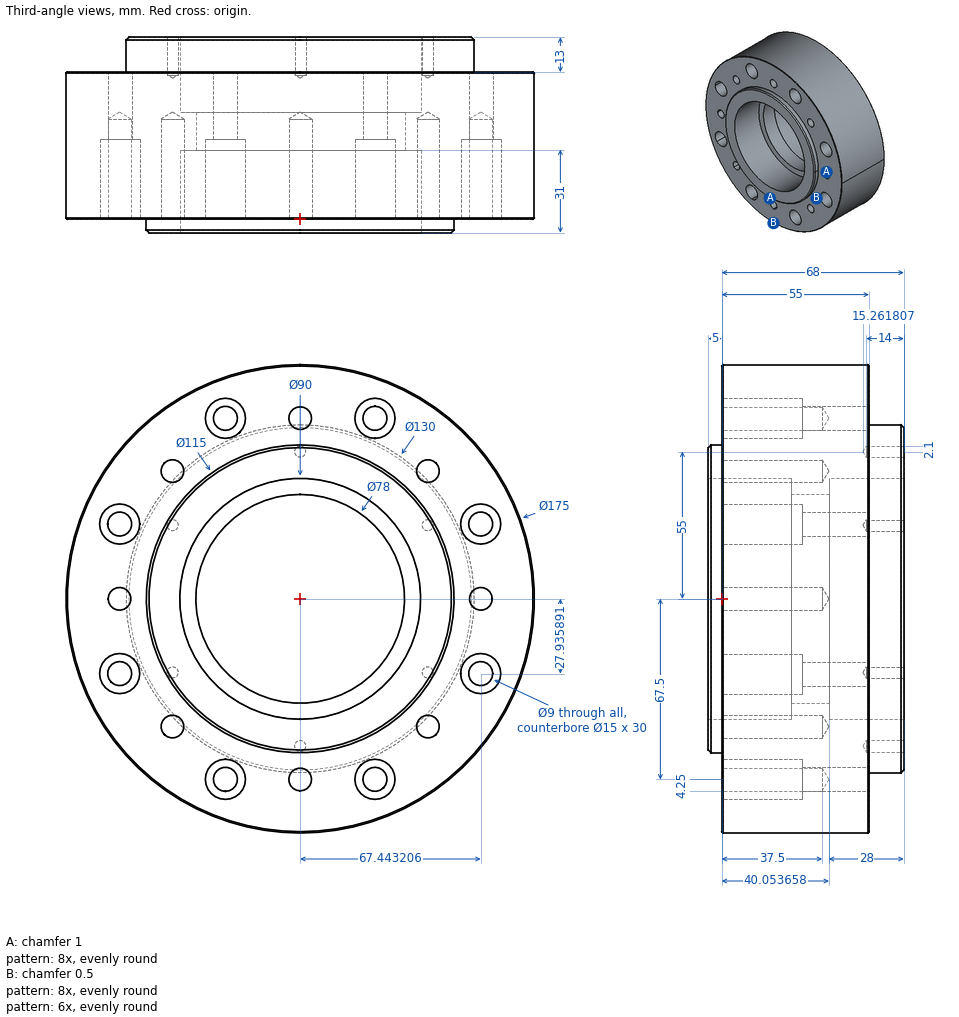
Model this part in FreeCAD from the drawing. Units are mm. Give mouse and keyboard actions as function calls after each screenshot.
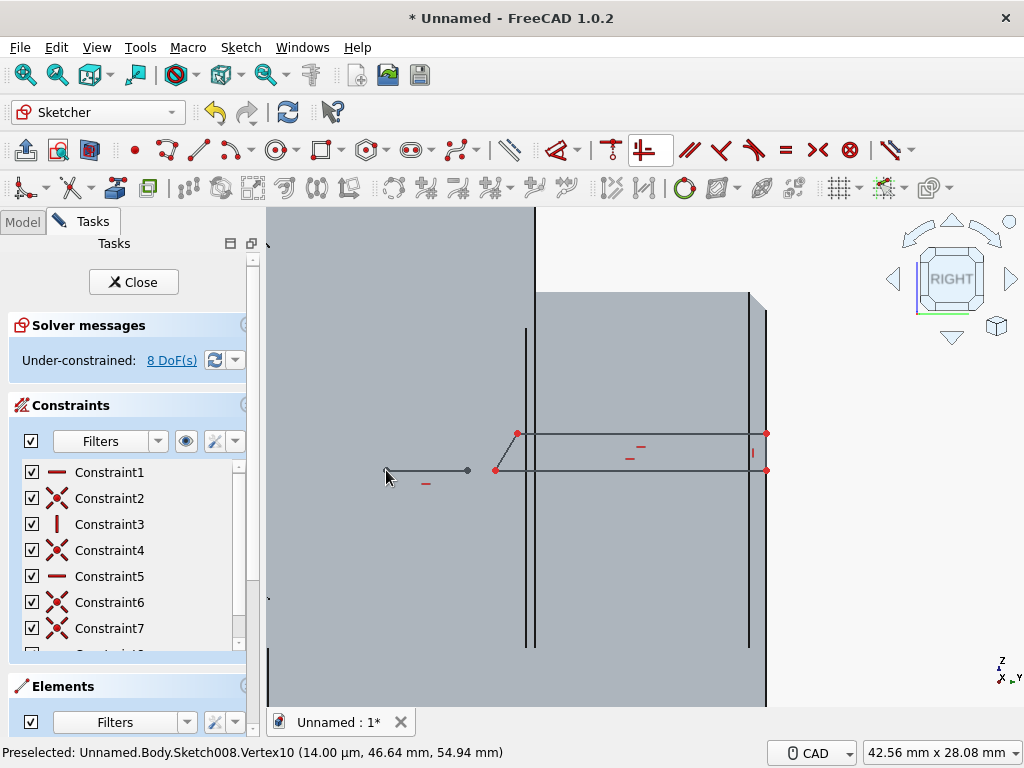
click(443, 471)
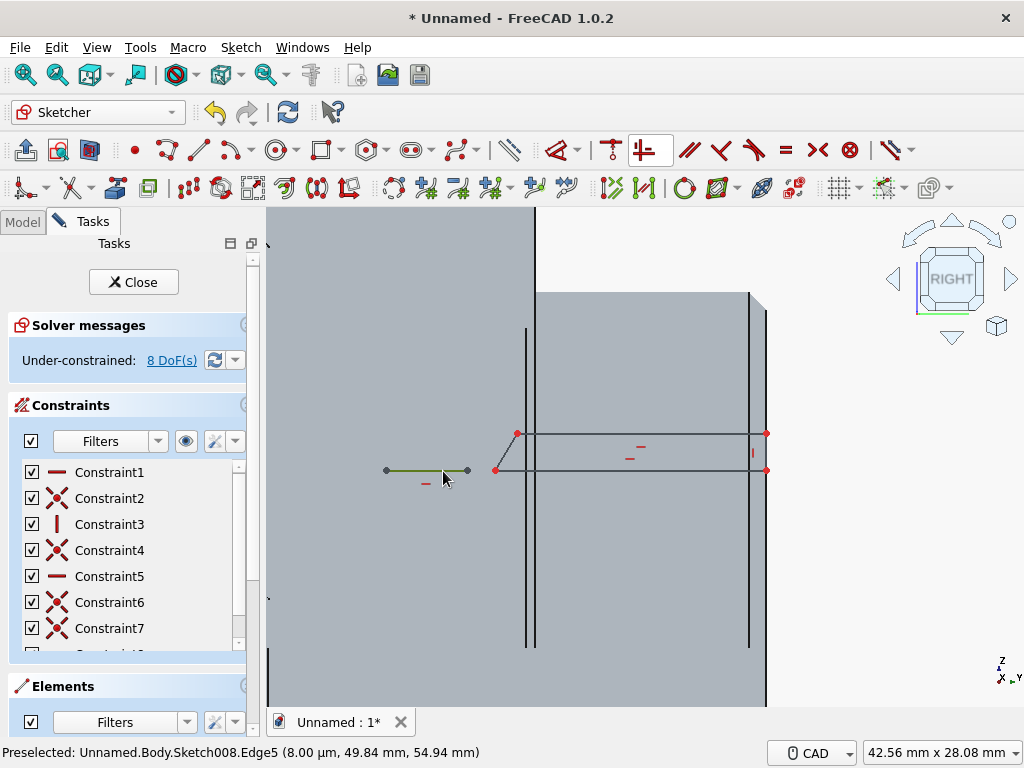
click(510, 150)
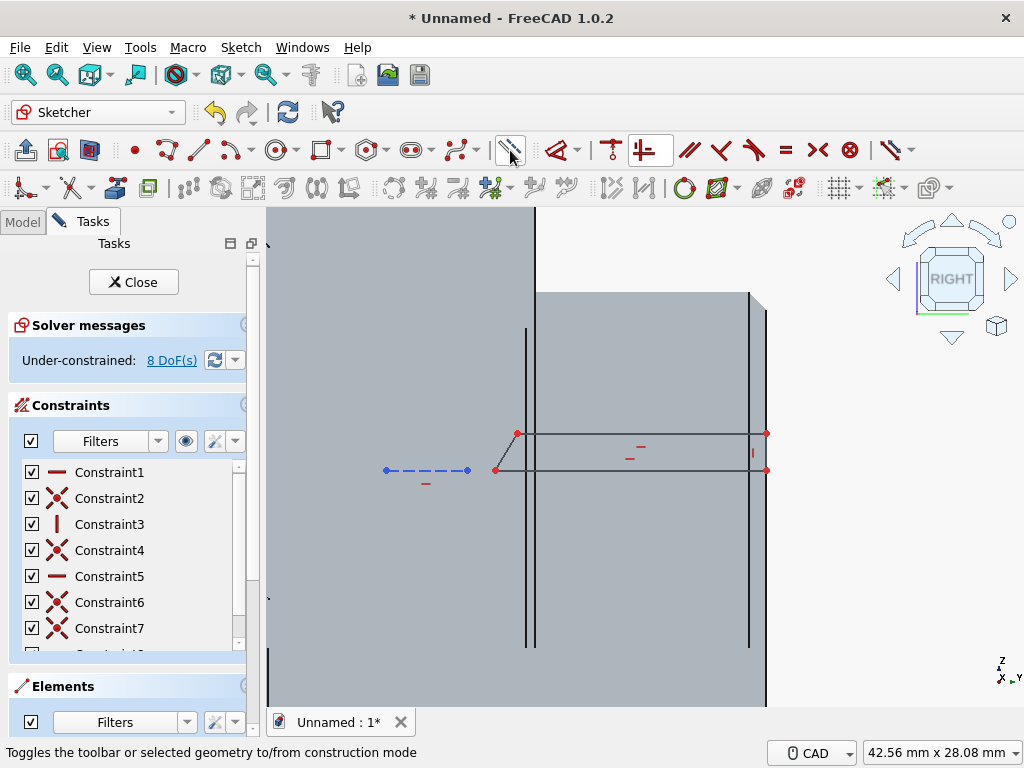
click(556, 150)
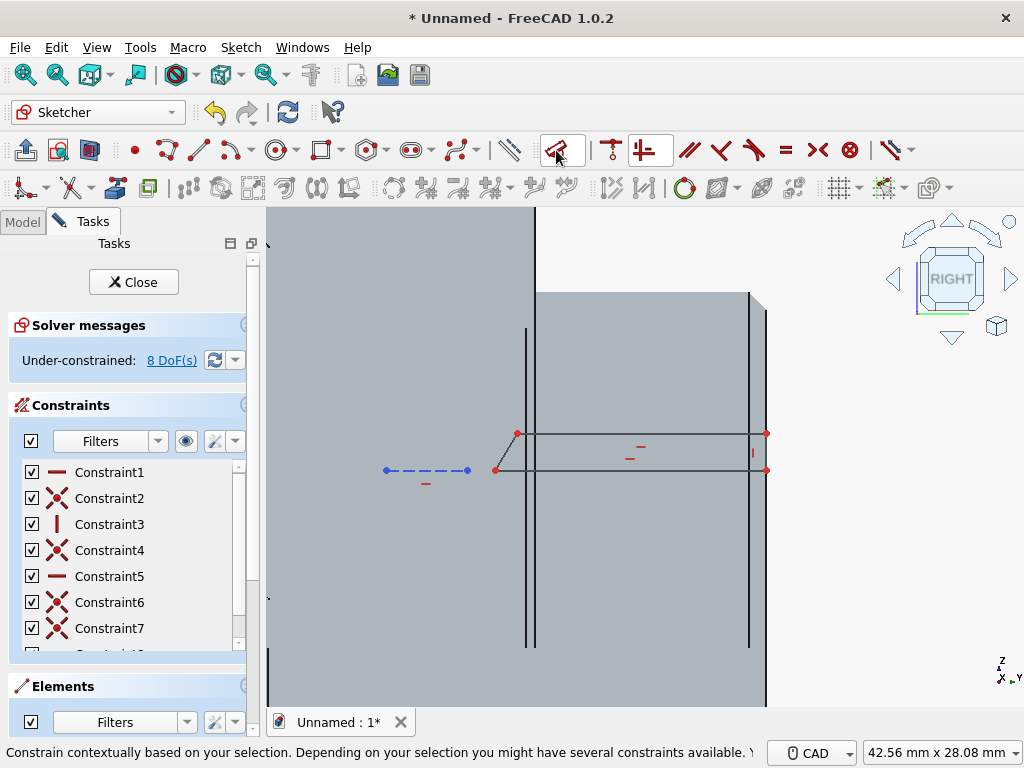
click(691, 434)
click(642, 400)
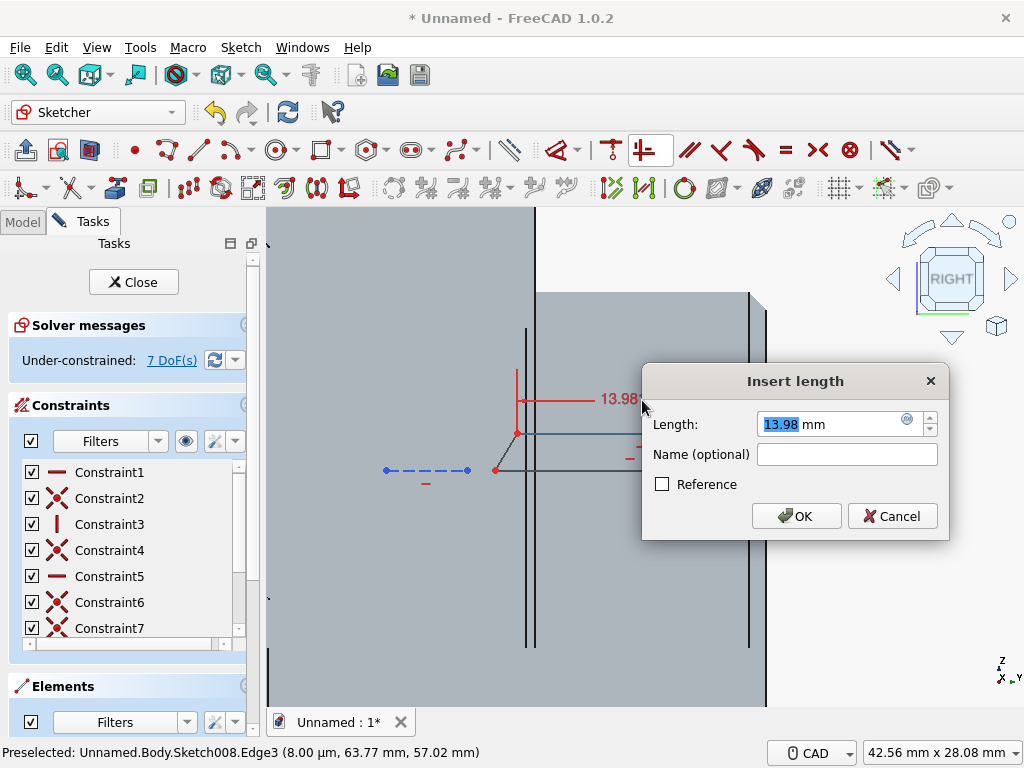
text(14)
key(Return)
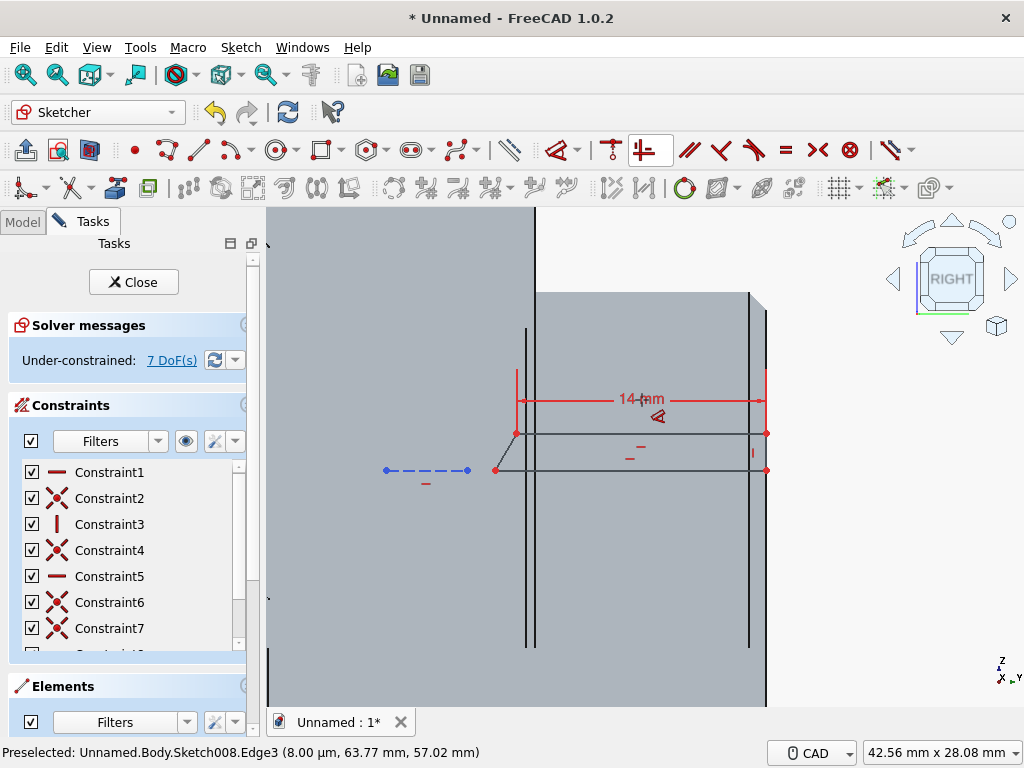
scroll(766, 460, up, 2)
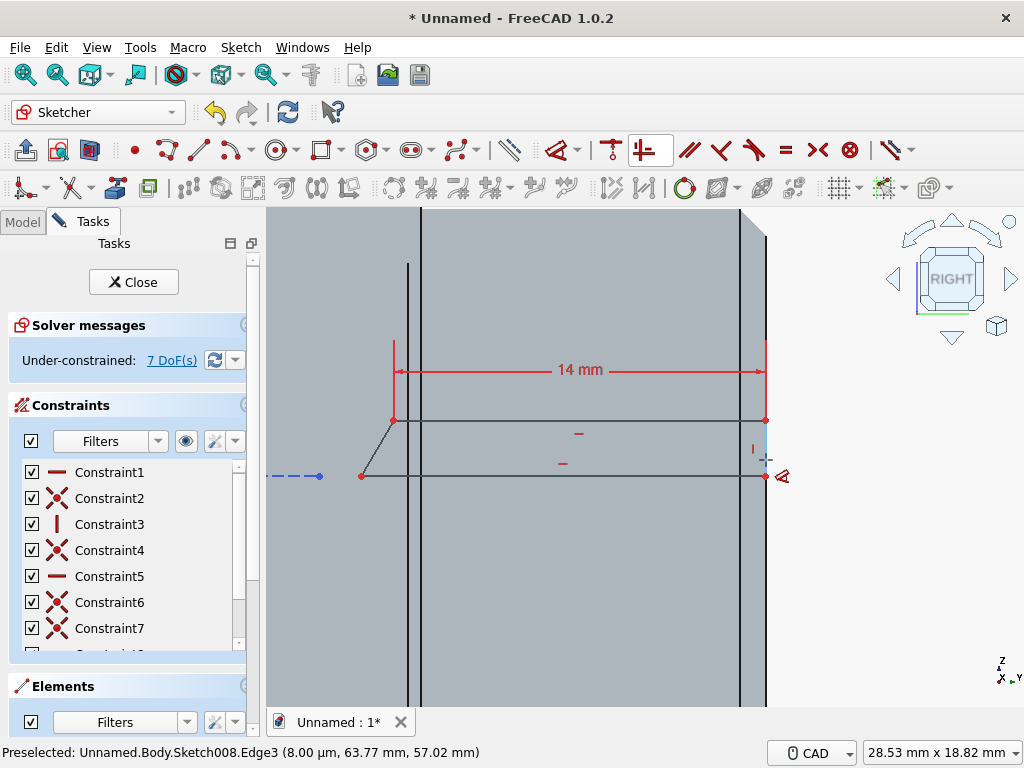
click(766, 460)
click(800, 449)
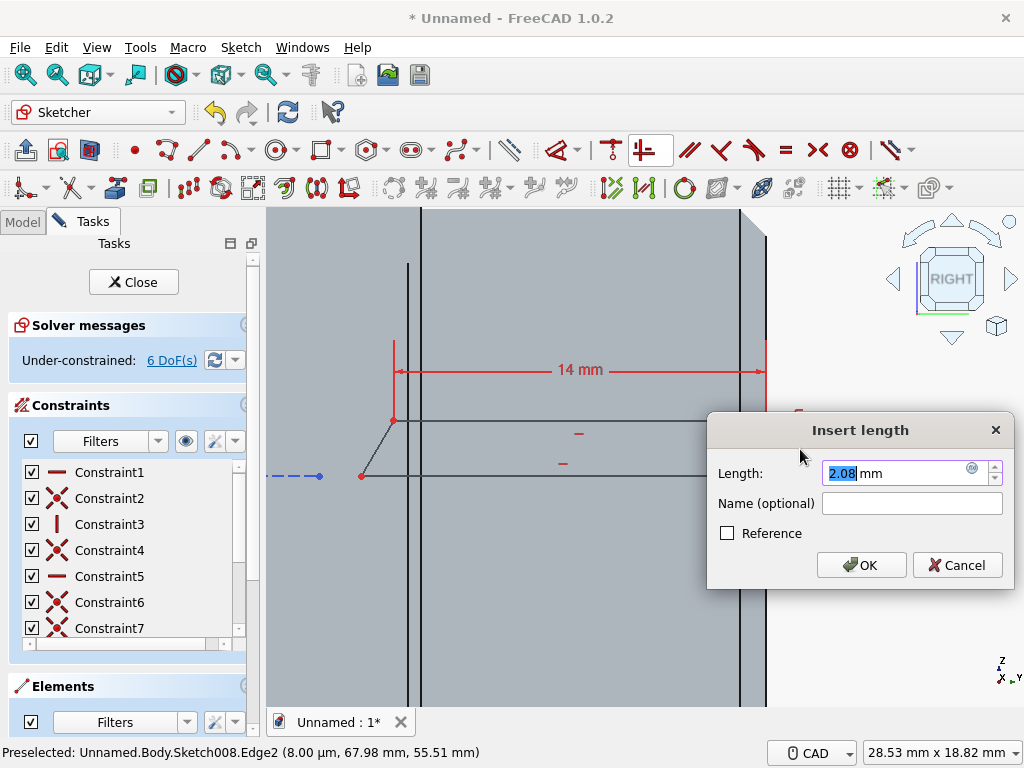
text(2.1)
key(Return)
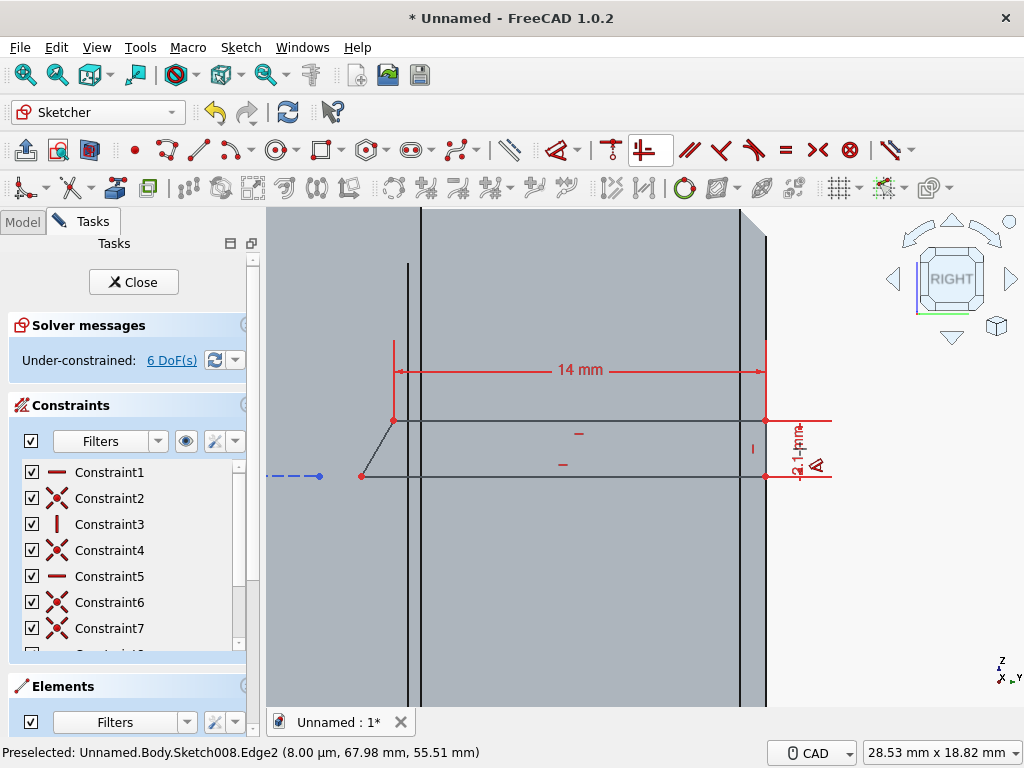
click(361, 477)
click(395, 578)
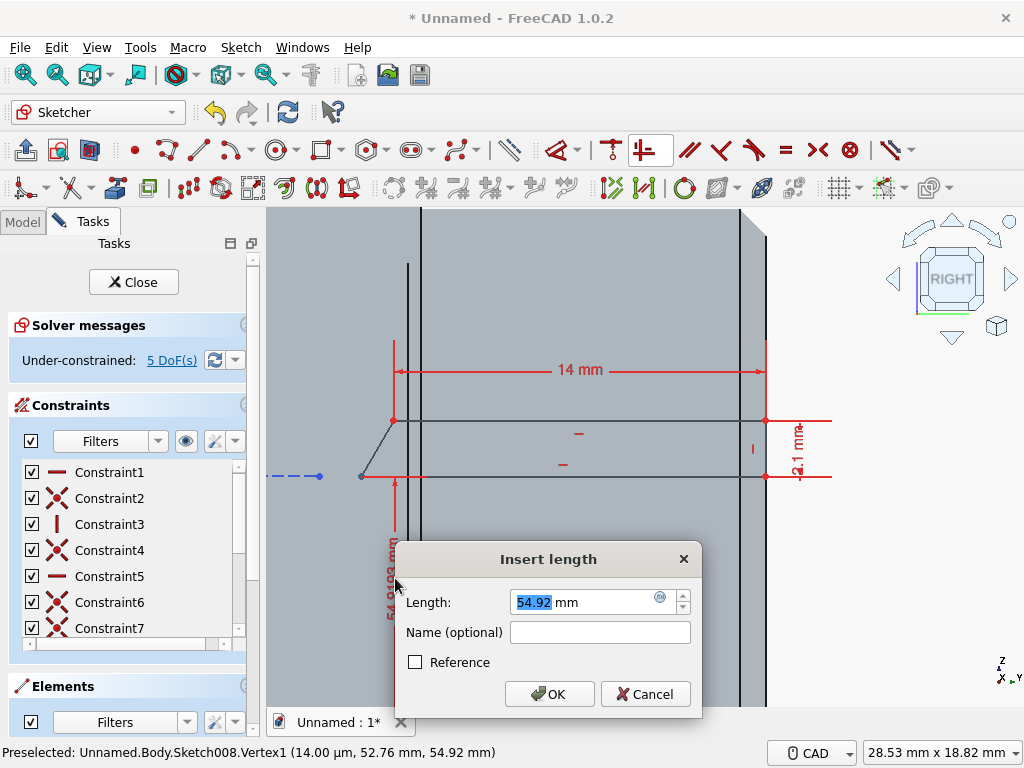
text(55)
key(Return)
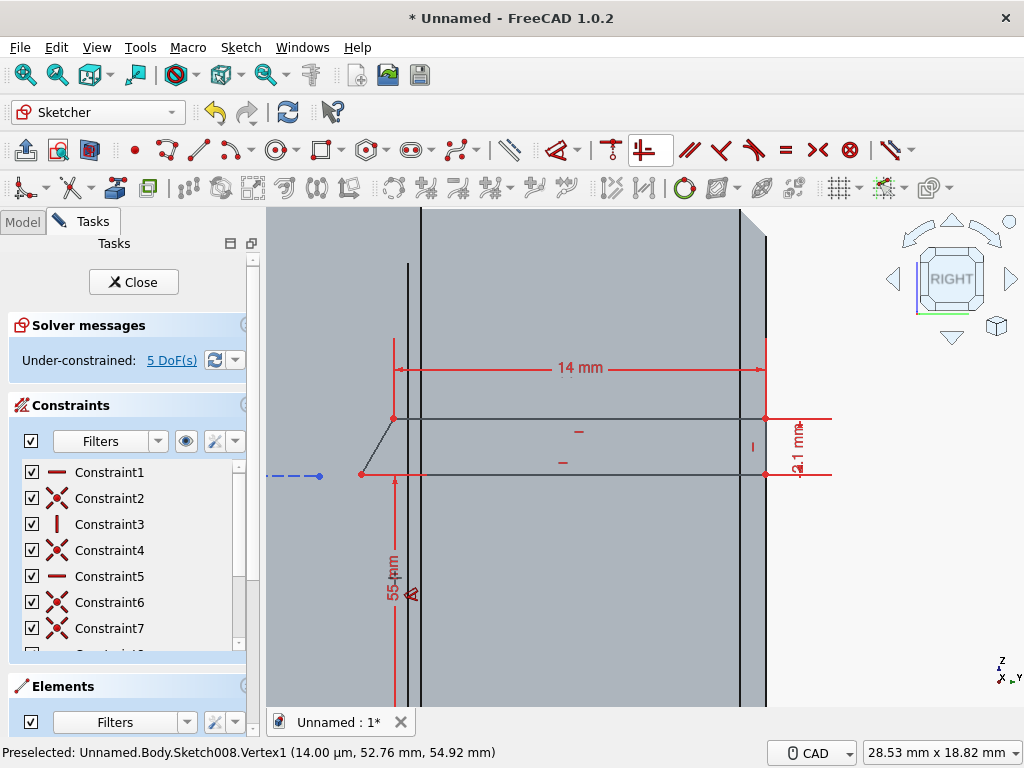
click(766, 475)
click(530, 441)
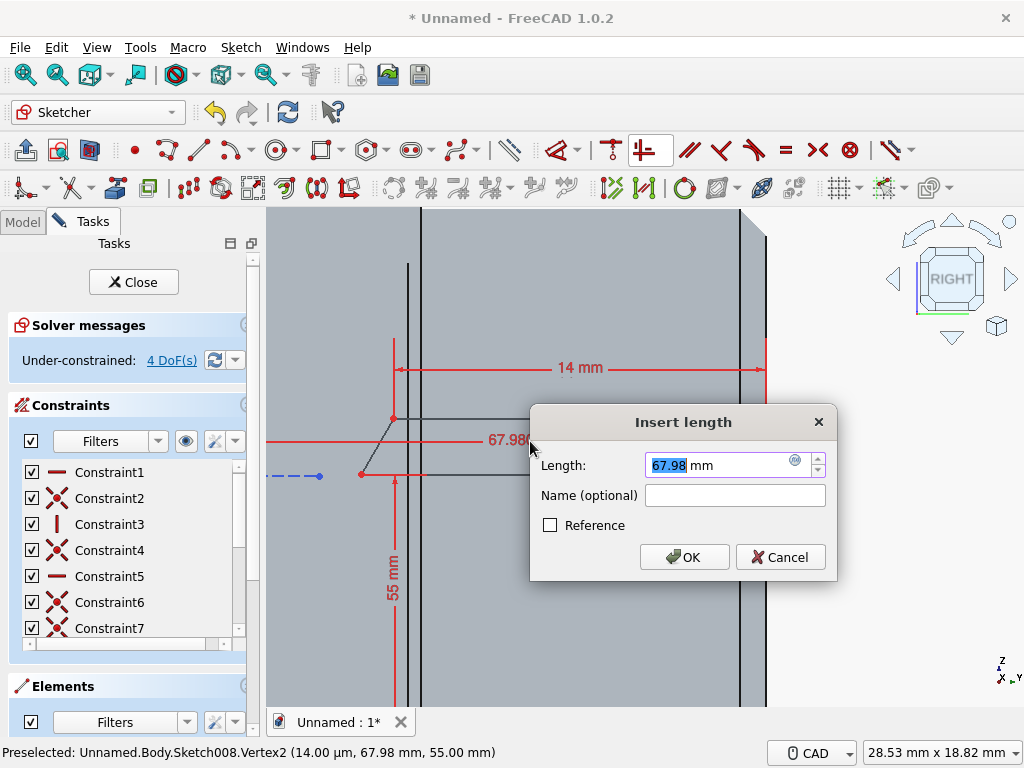
text(68)
key(Return)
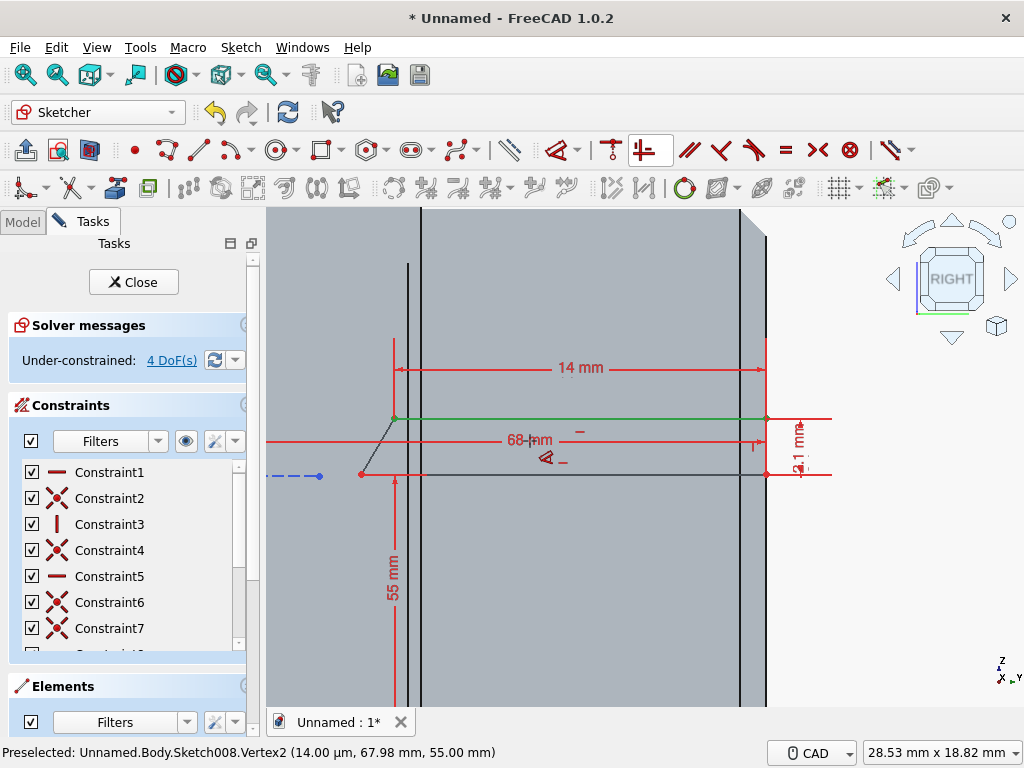
click(320, 476)
click(354, 531)